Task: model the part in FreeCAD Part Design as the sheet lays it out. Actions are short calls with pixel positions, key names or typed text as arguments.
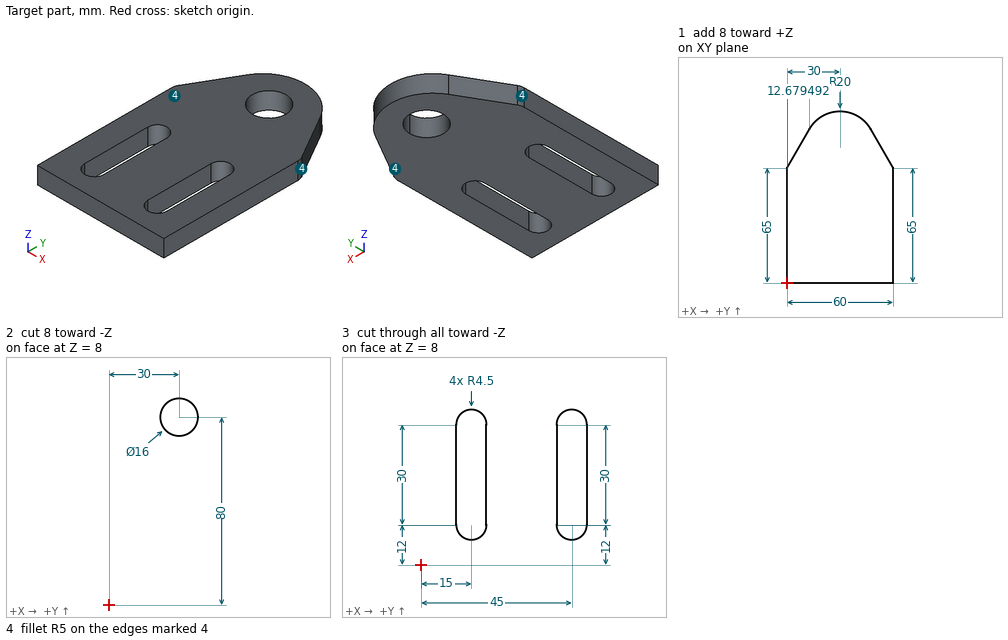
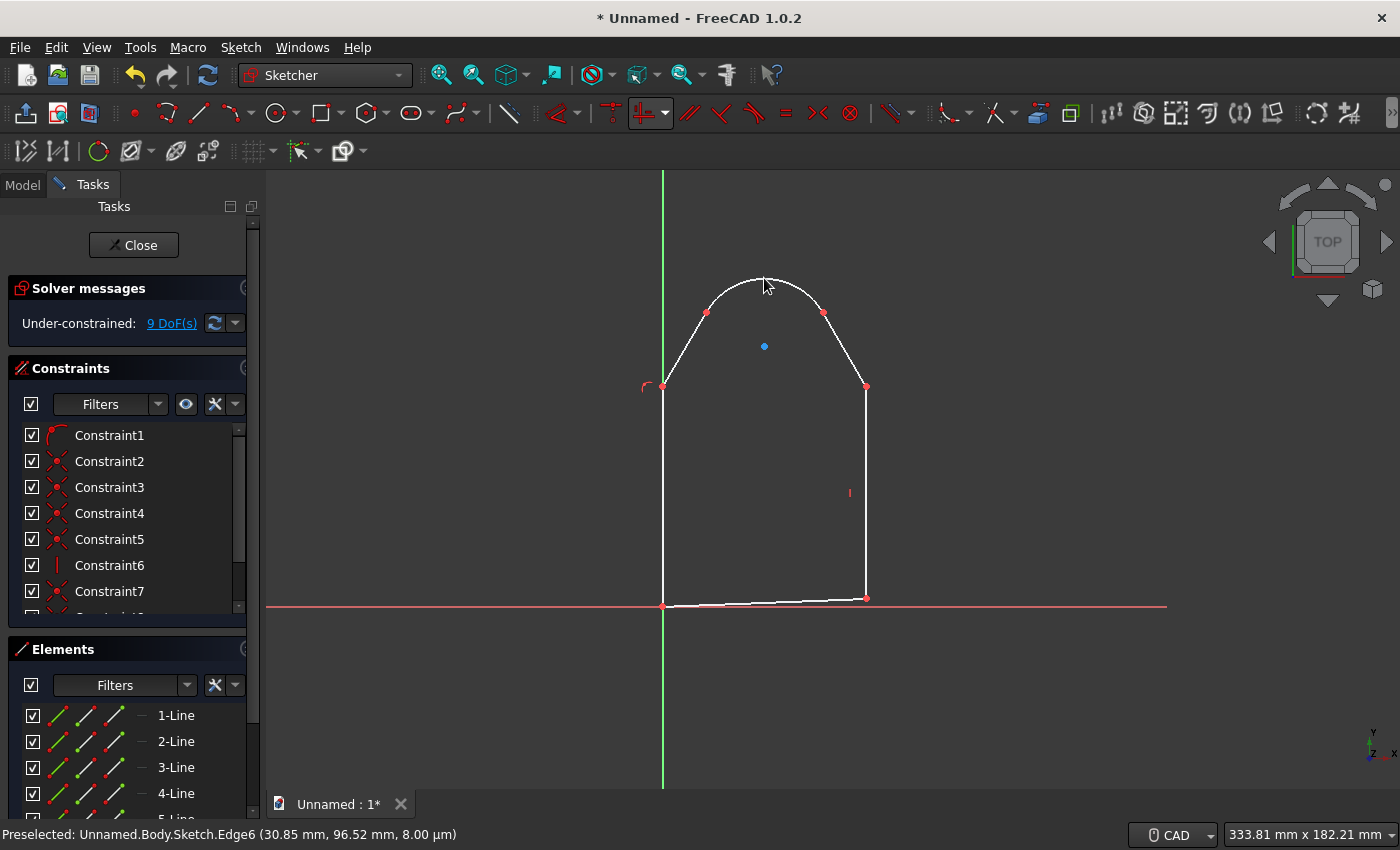
click(693, 335)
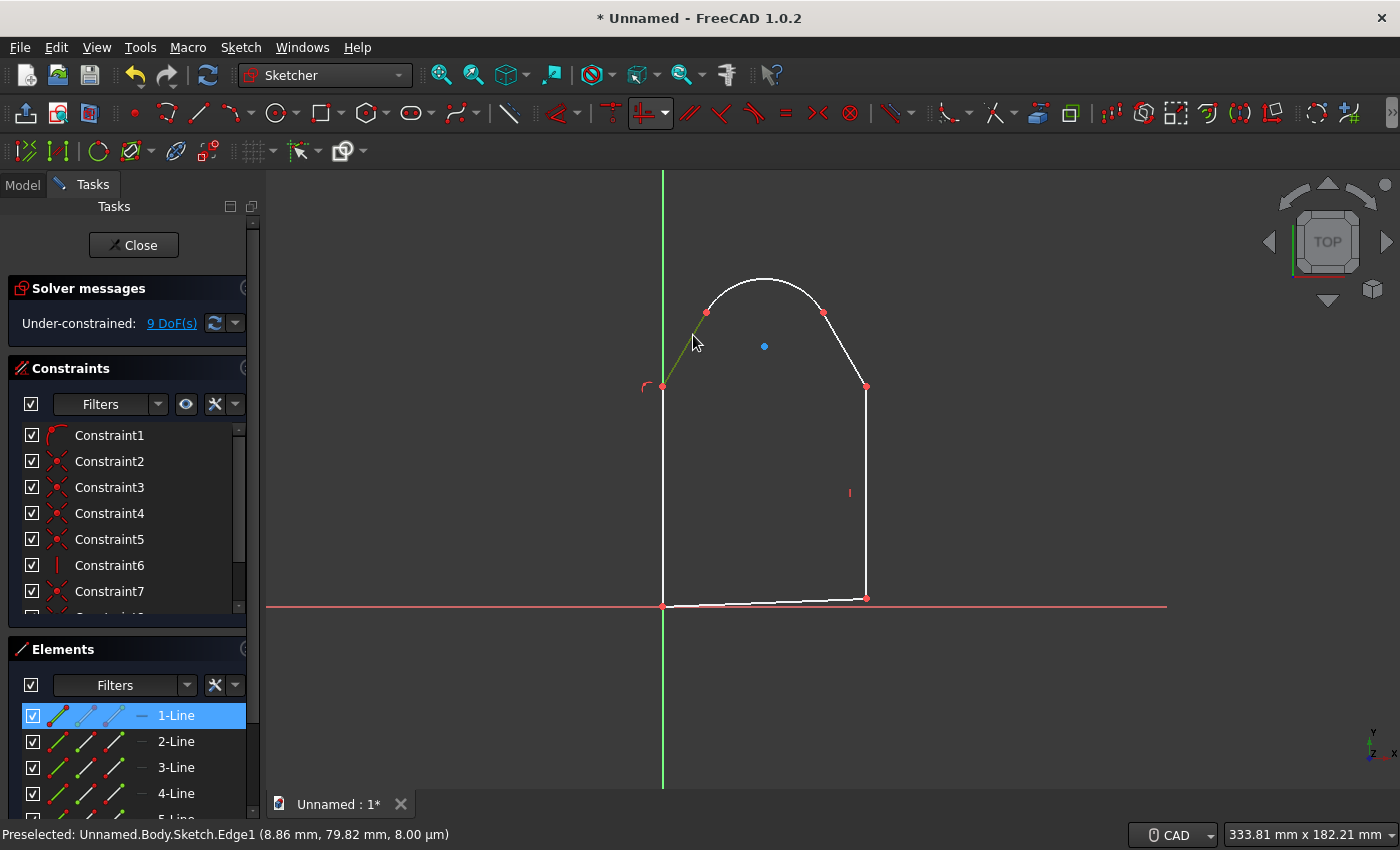
click(792, 285)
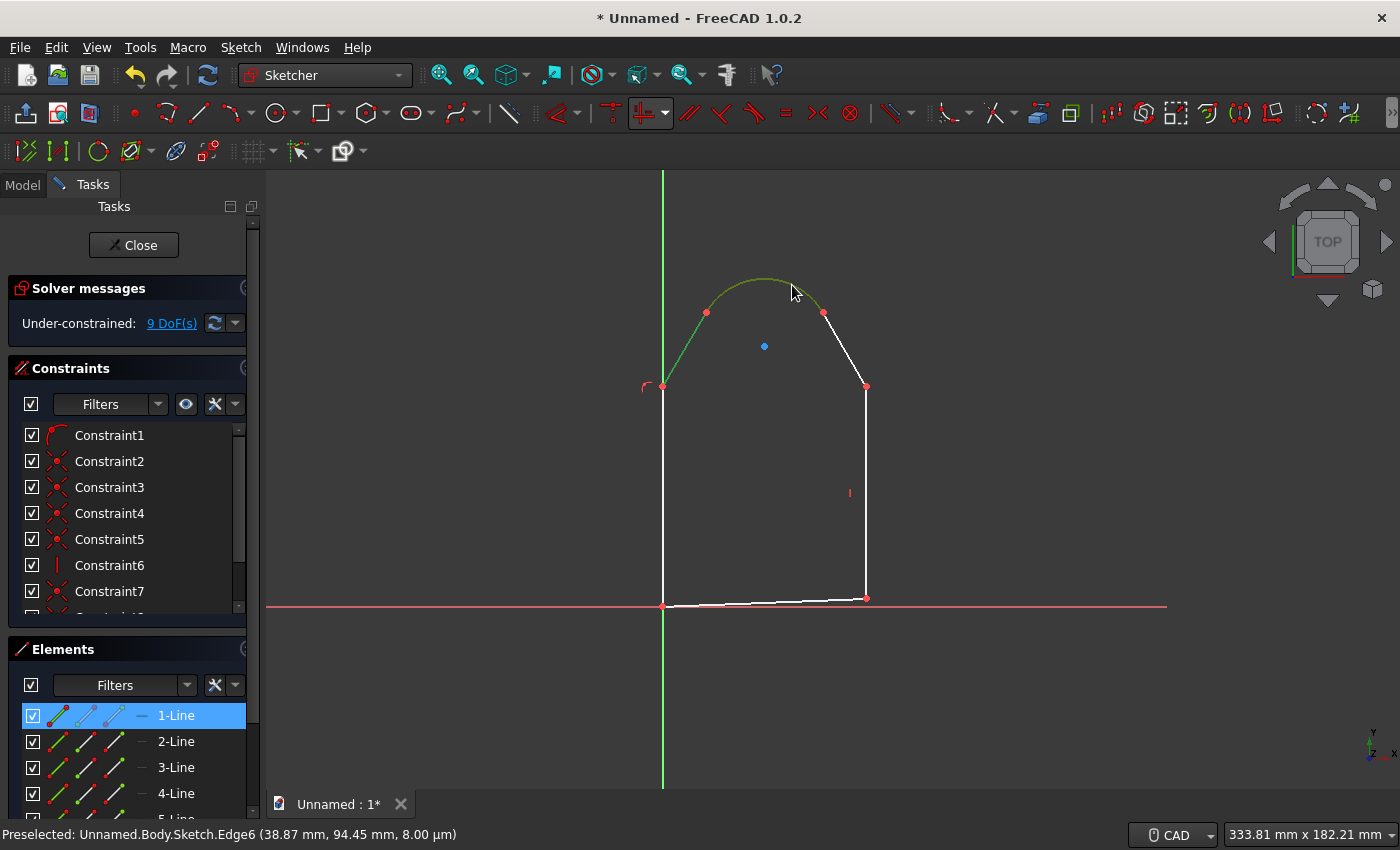
click(754, 114)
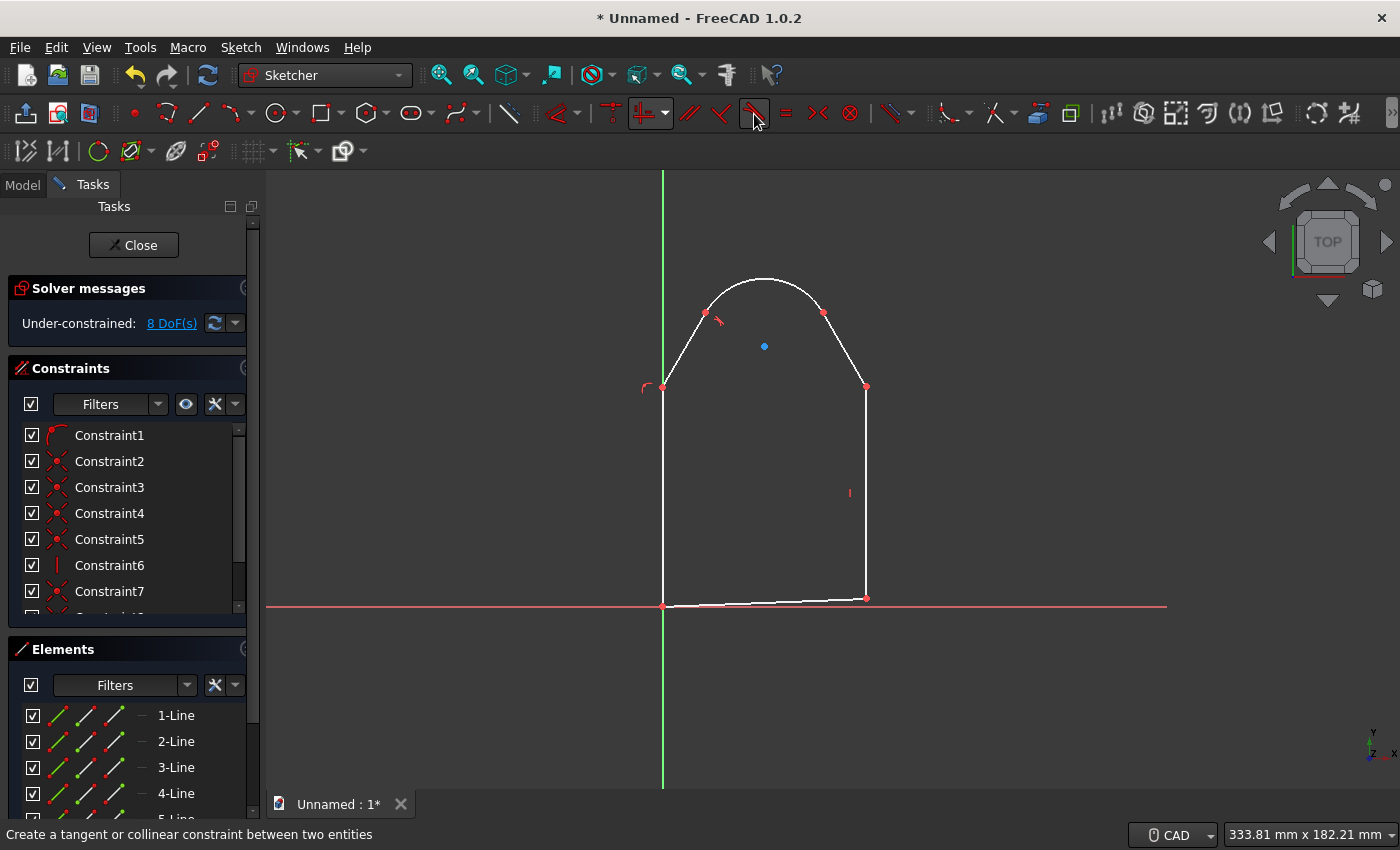
click(853, 365)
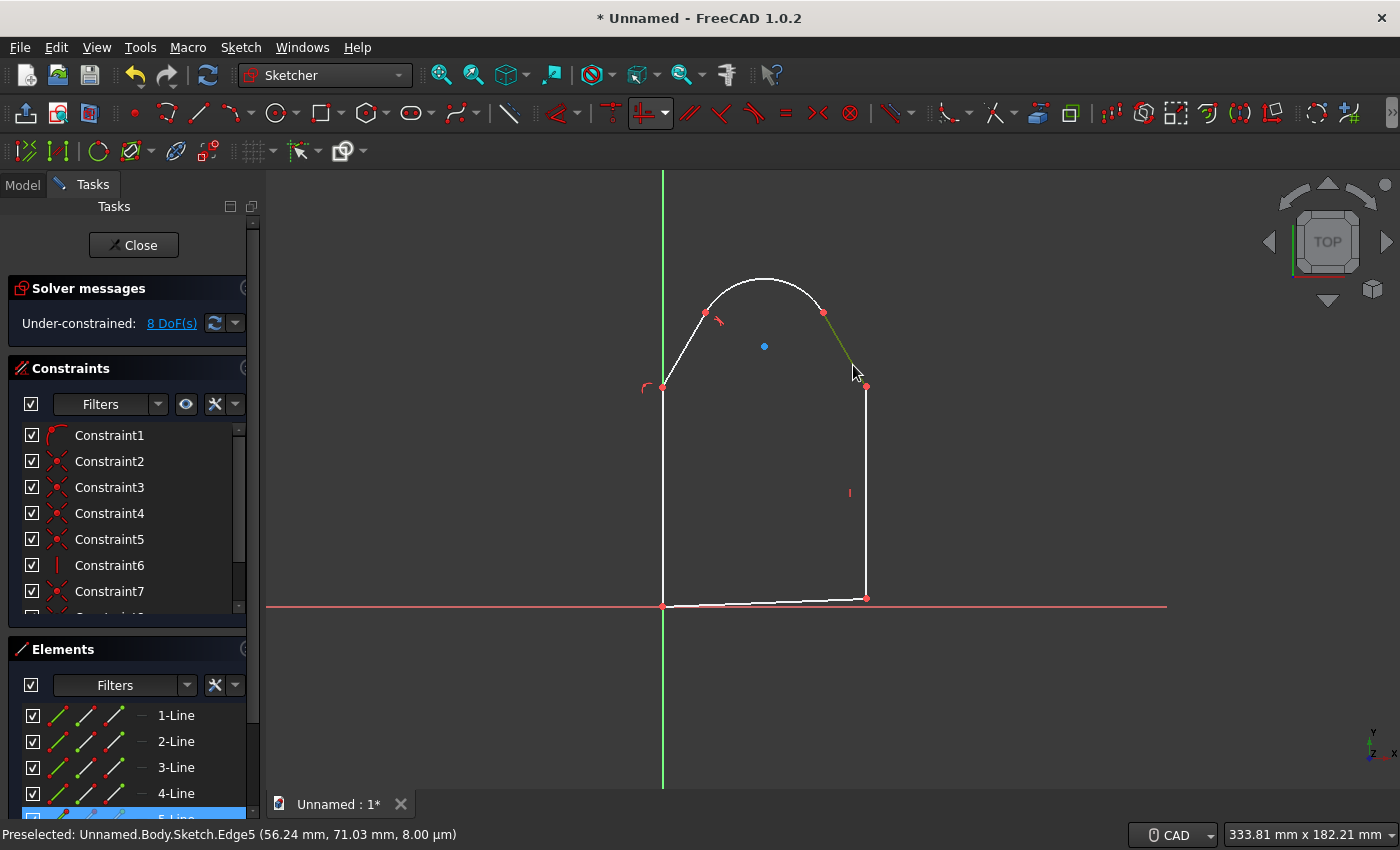
click(792, 285)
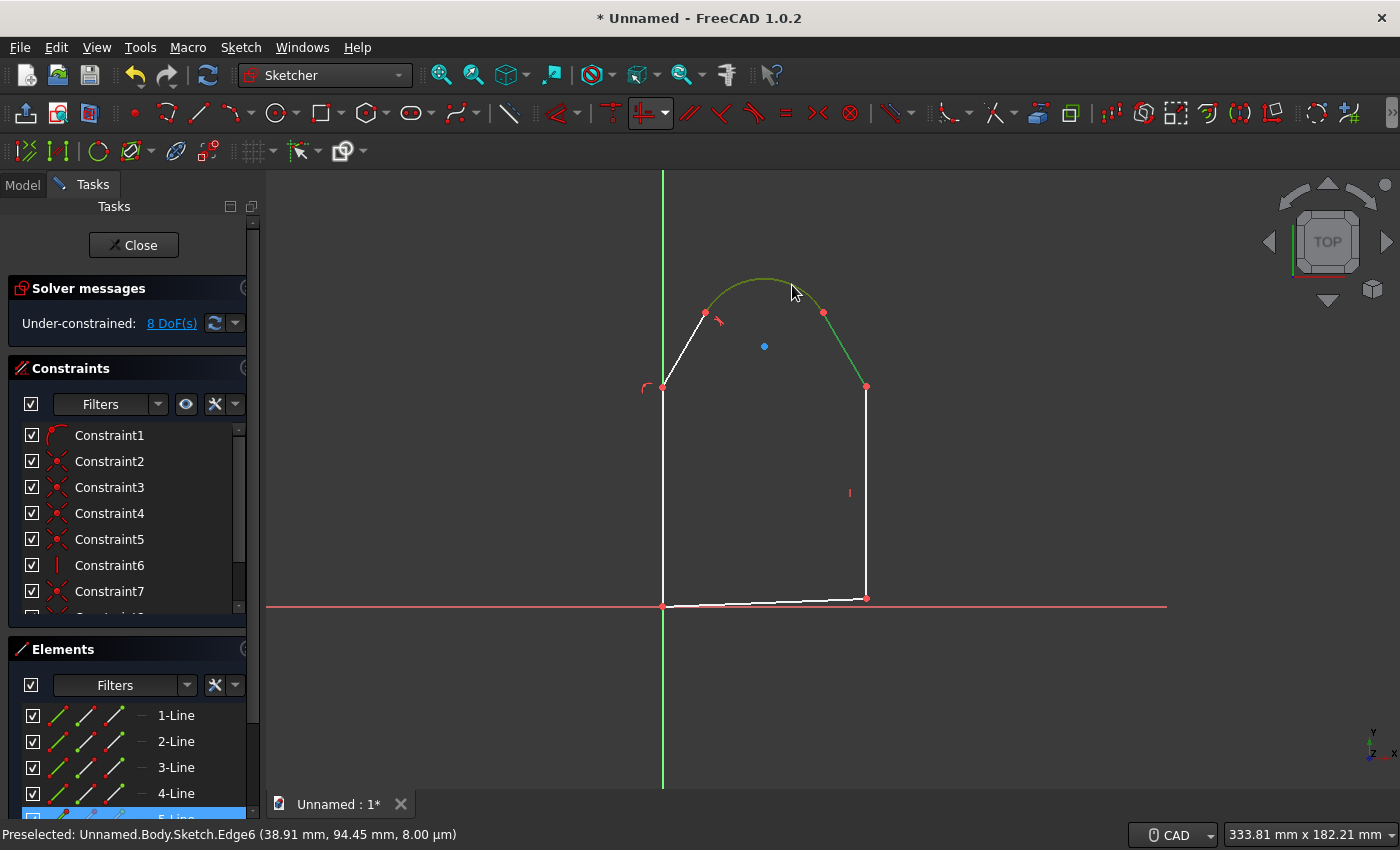
key(t)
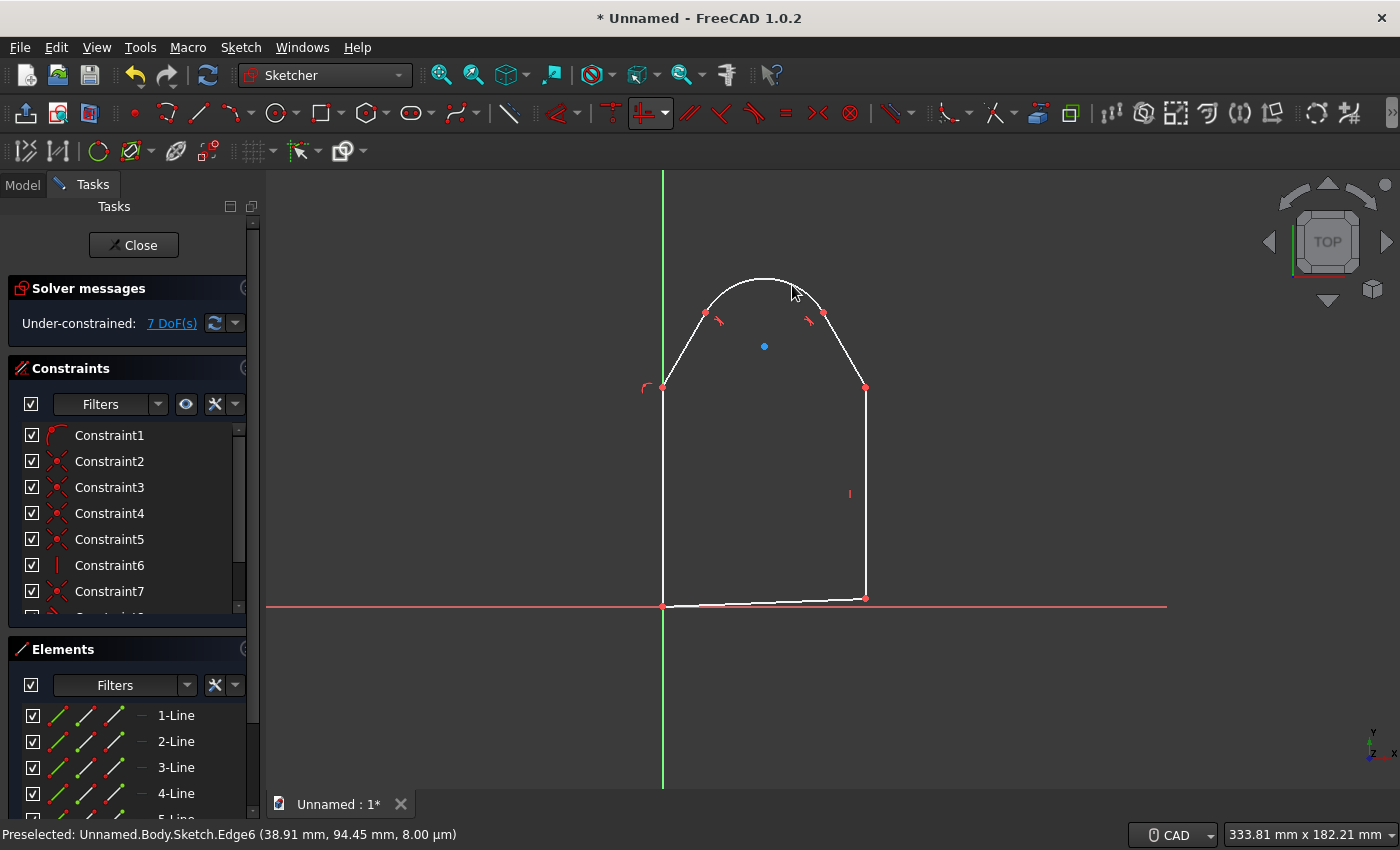
click(724, 605)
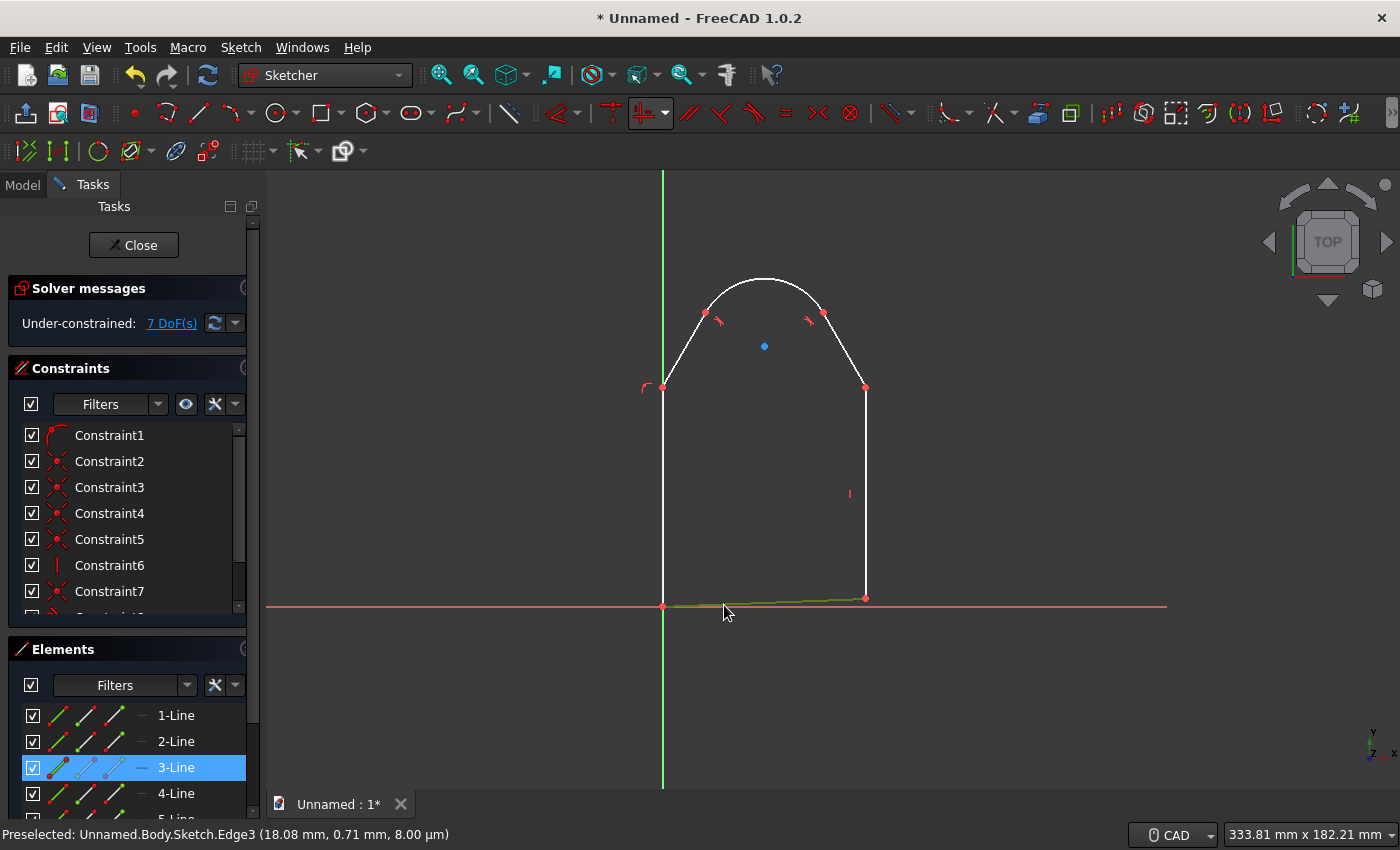
key(h)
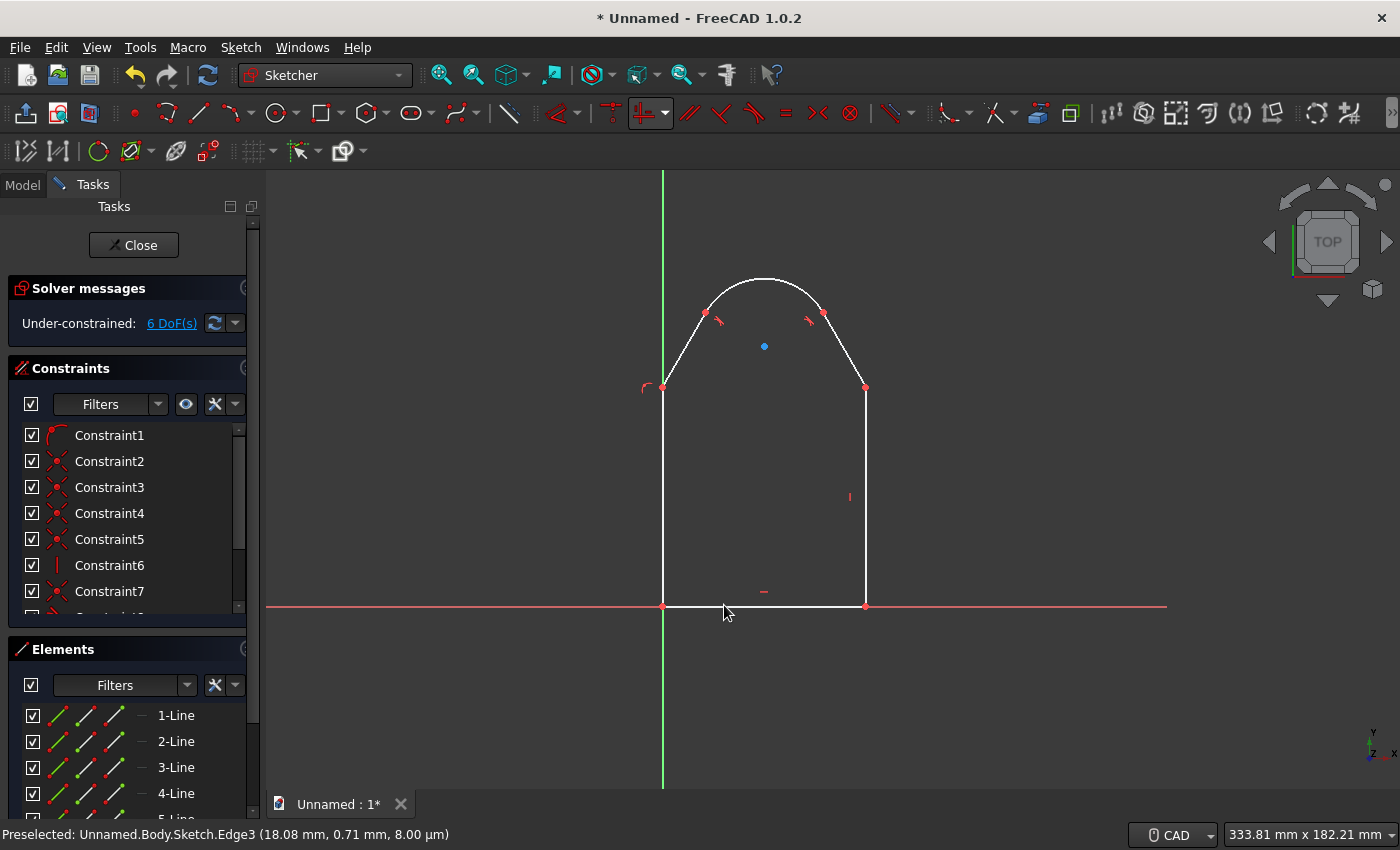
click(556, 114)